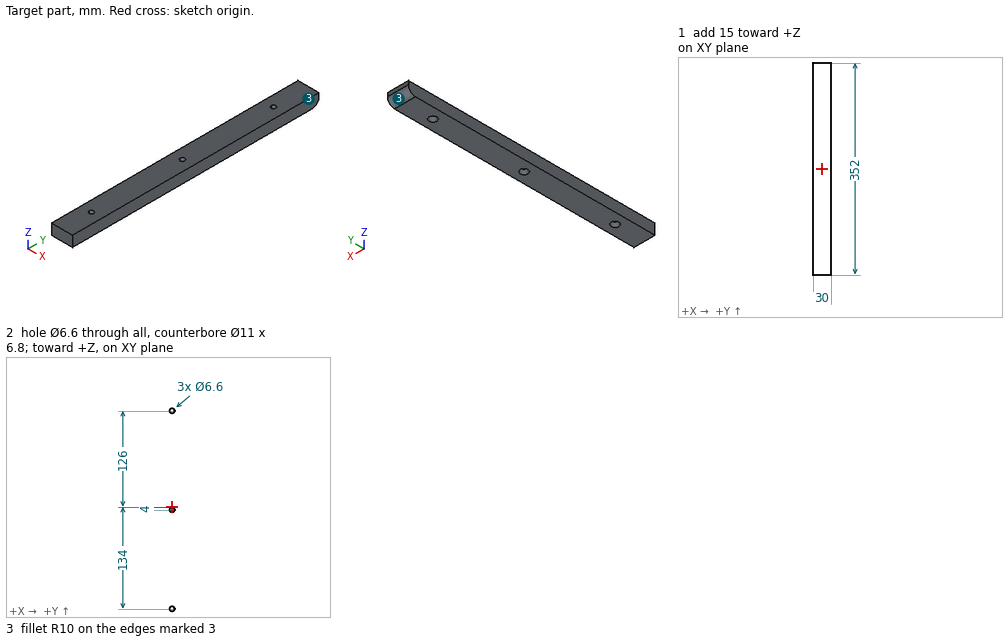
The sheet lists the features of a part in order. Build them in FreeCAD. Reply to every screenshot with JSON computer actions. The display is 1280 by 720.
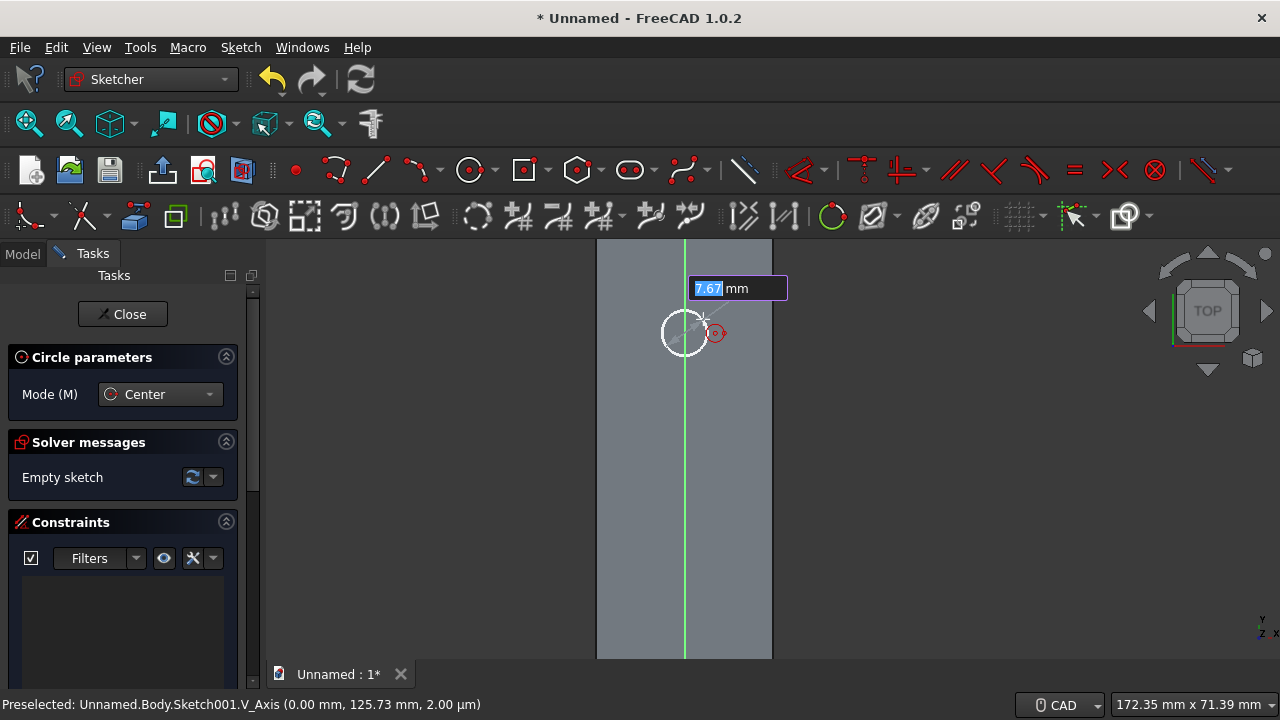
{"action": "type", "text": "6.6"}
{"action": "key", "text": "Return"}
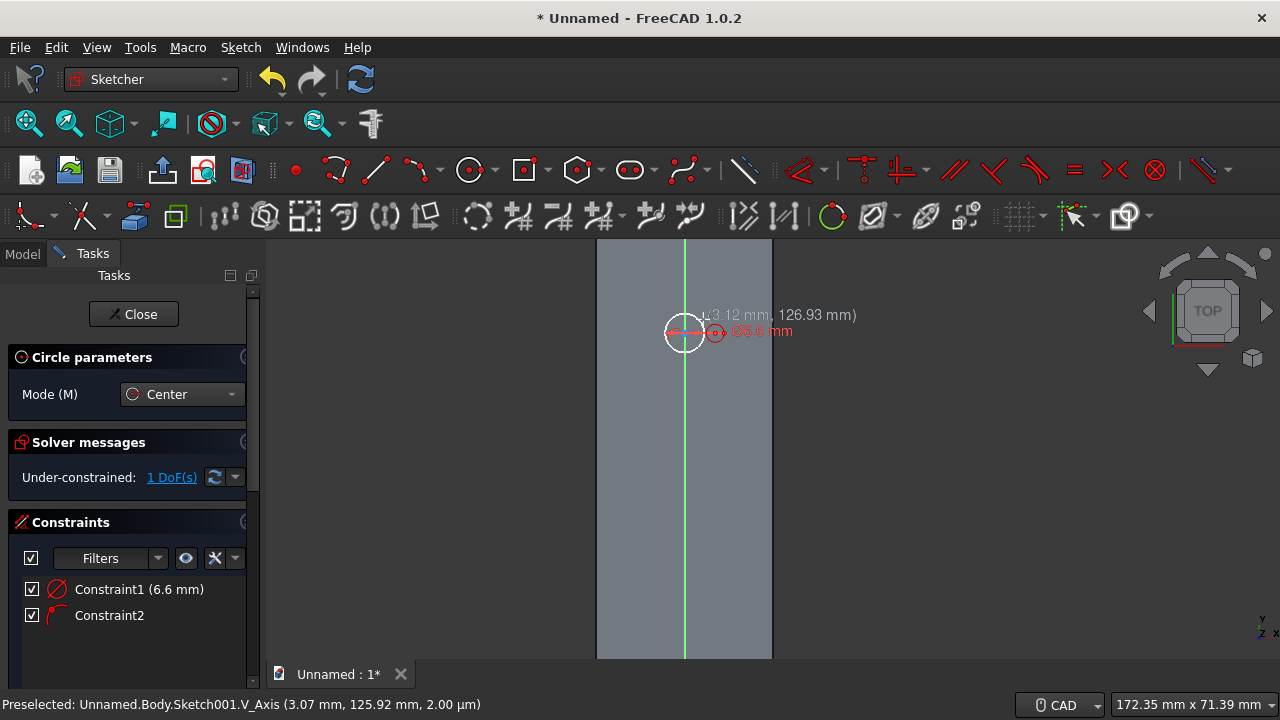
{"action": "scroll", "coordinate": [708, 322], "scroll_direction": "down", "scroll_amount": 9}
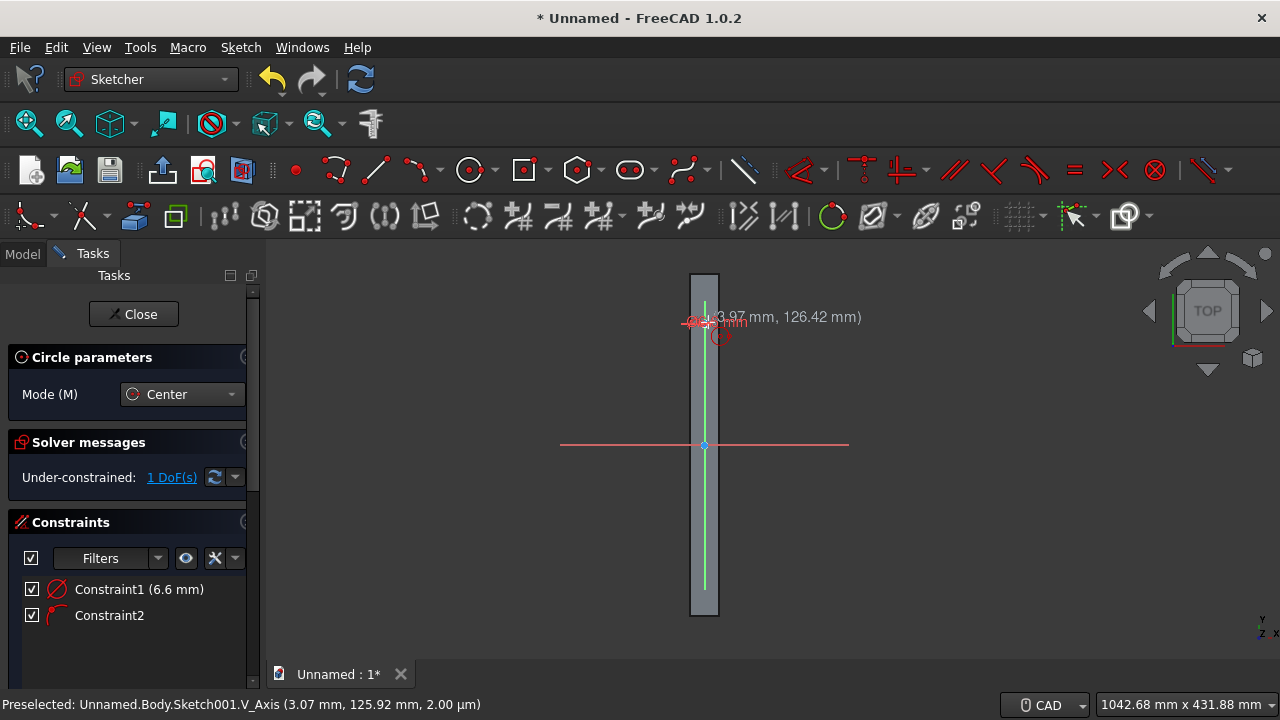
{"action": "scroll", "coordinate": [705, 449], "scroll_direction": "up", "scroll_amount": 10}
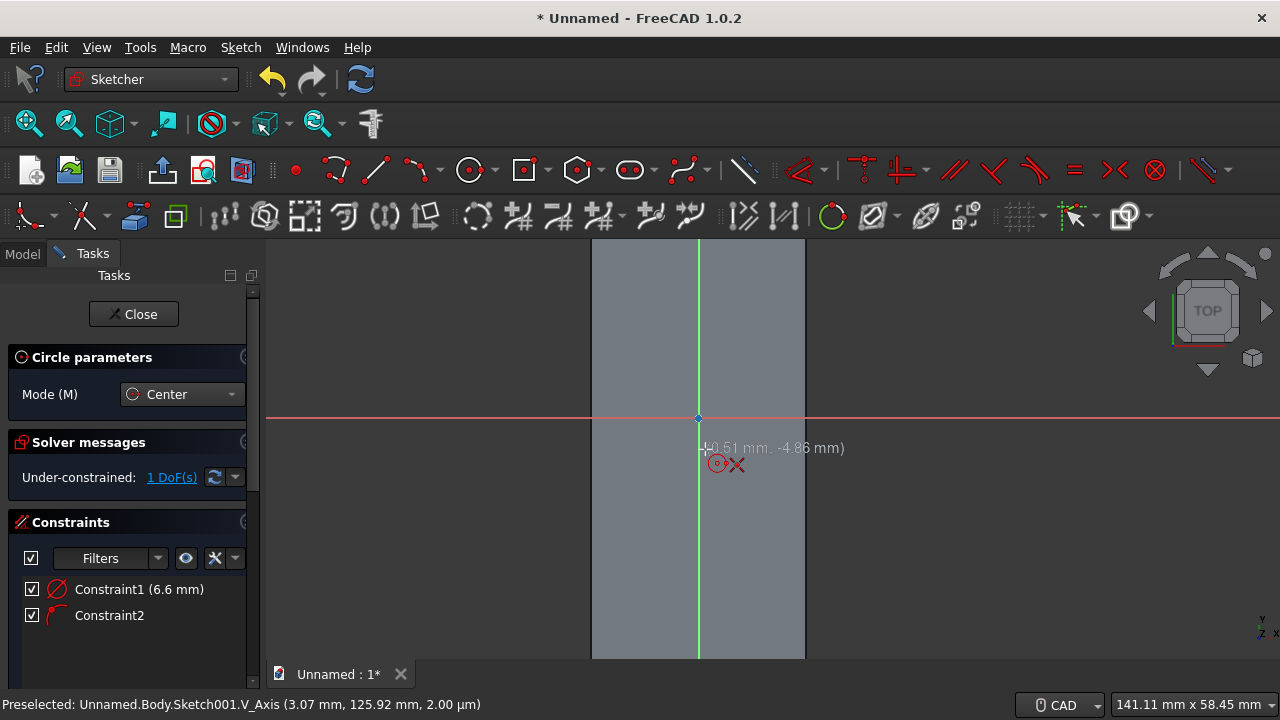
{"action": "left_click", "coordinate": [699, 447]}
{"action": "mouse_move", "coordinate": [715, 464]}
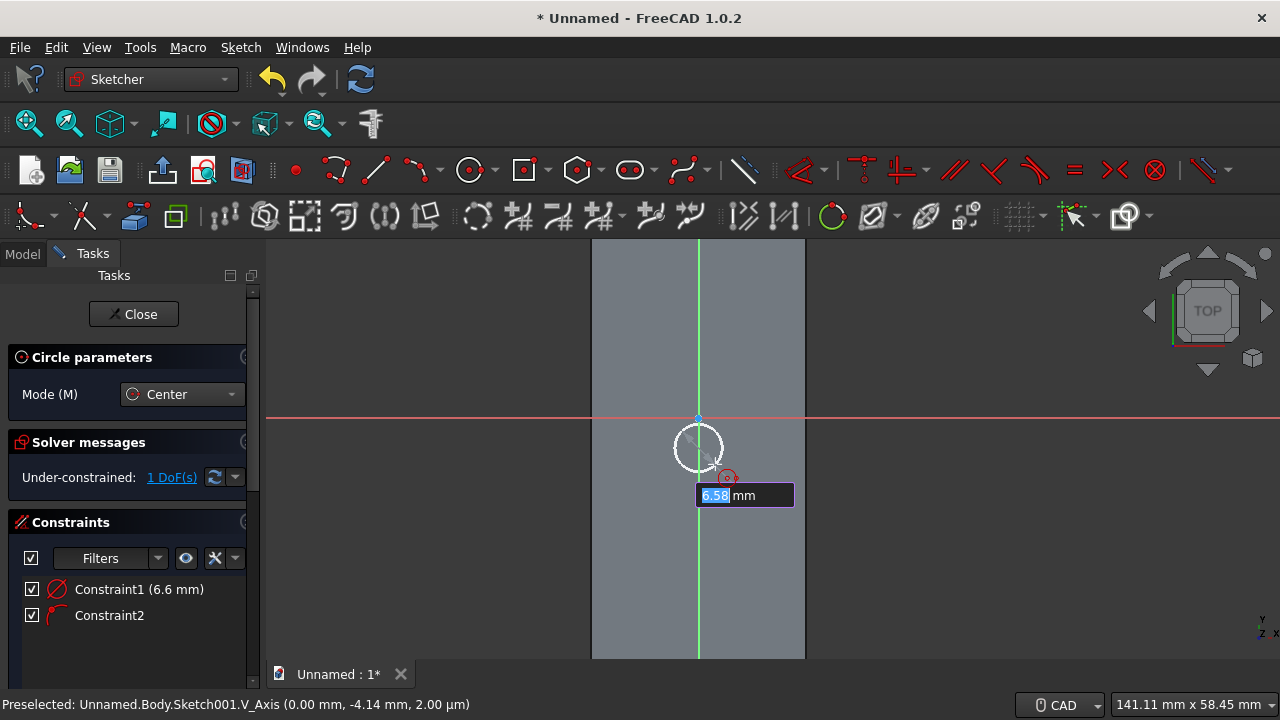
{"action": "type", "text": "6.6"}
{"action": "key", "text": "Return"}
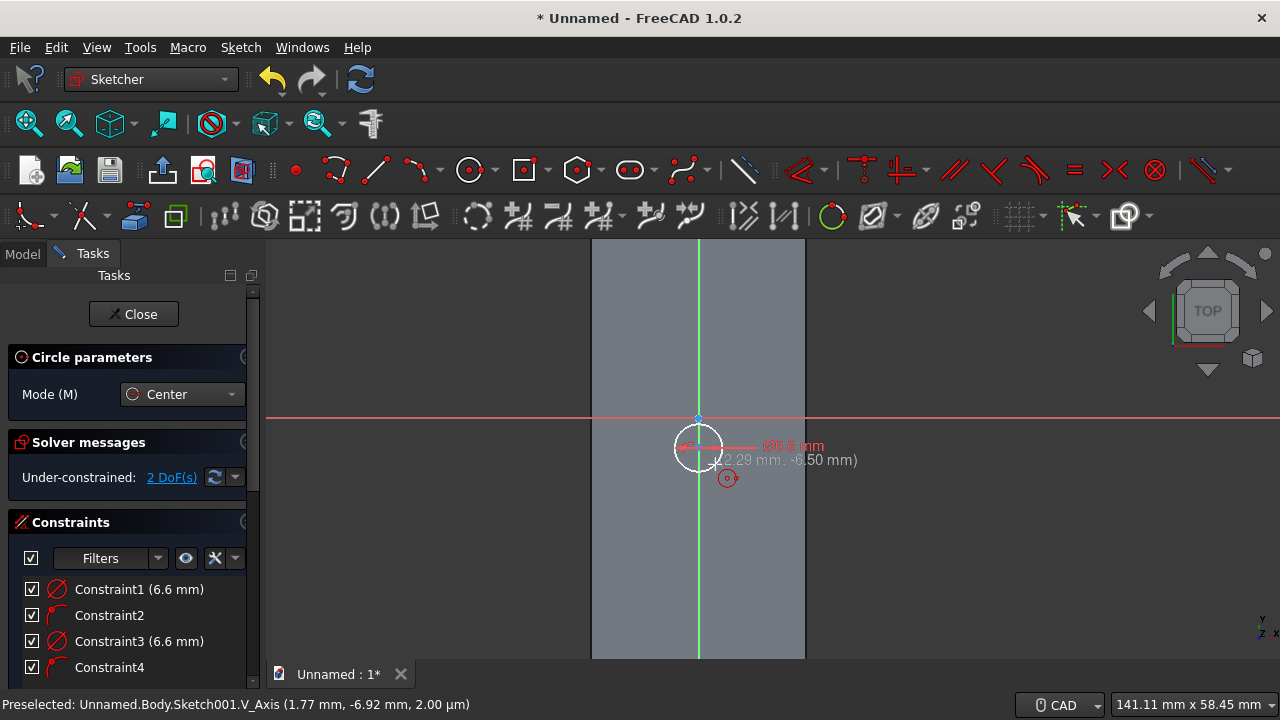
{"action": "scroll", "coordinate": [705, 449], "scroll_direction": "down", "scroll_amount": 10}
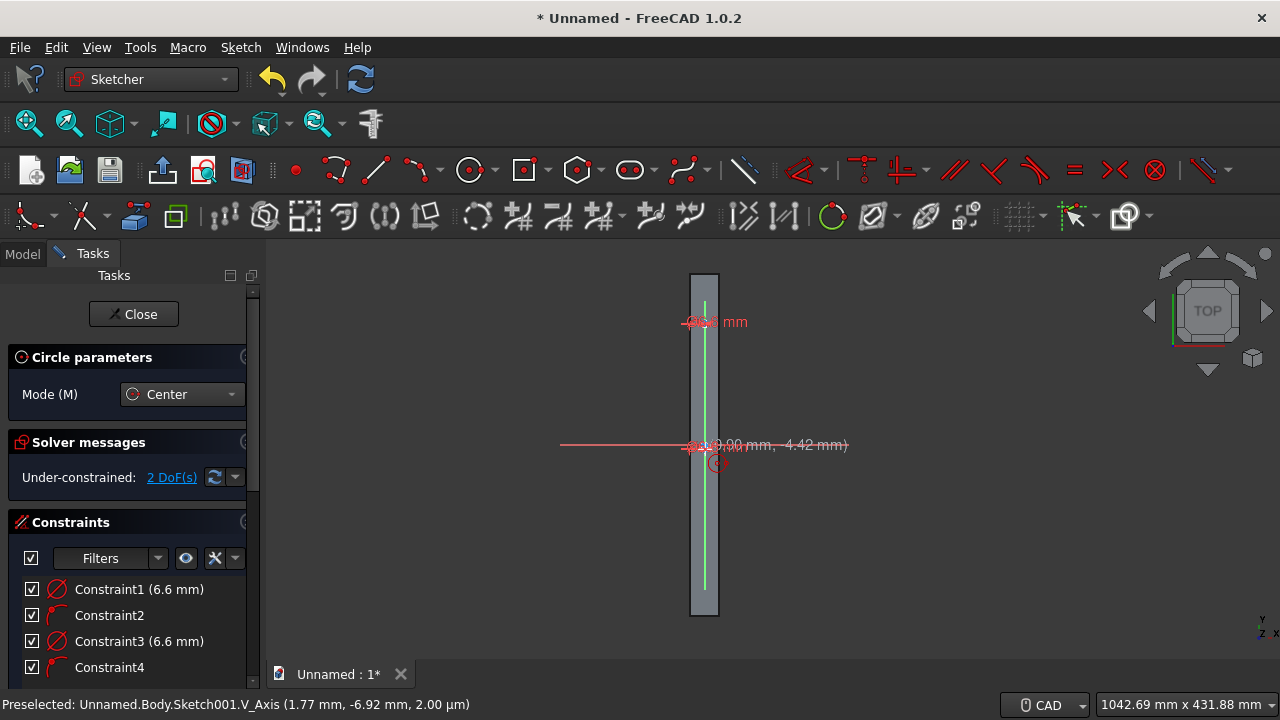
{"action": "scroll", "coordinate": [705, 576], "scroll_direction": "up", "scroll_amount": 10}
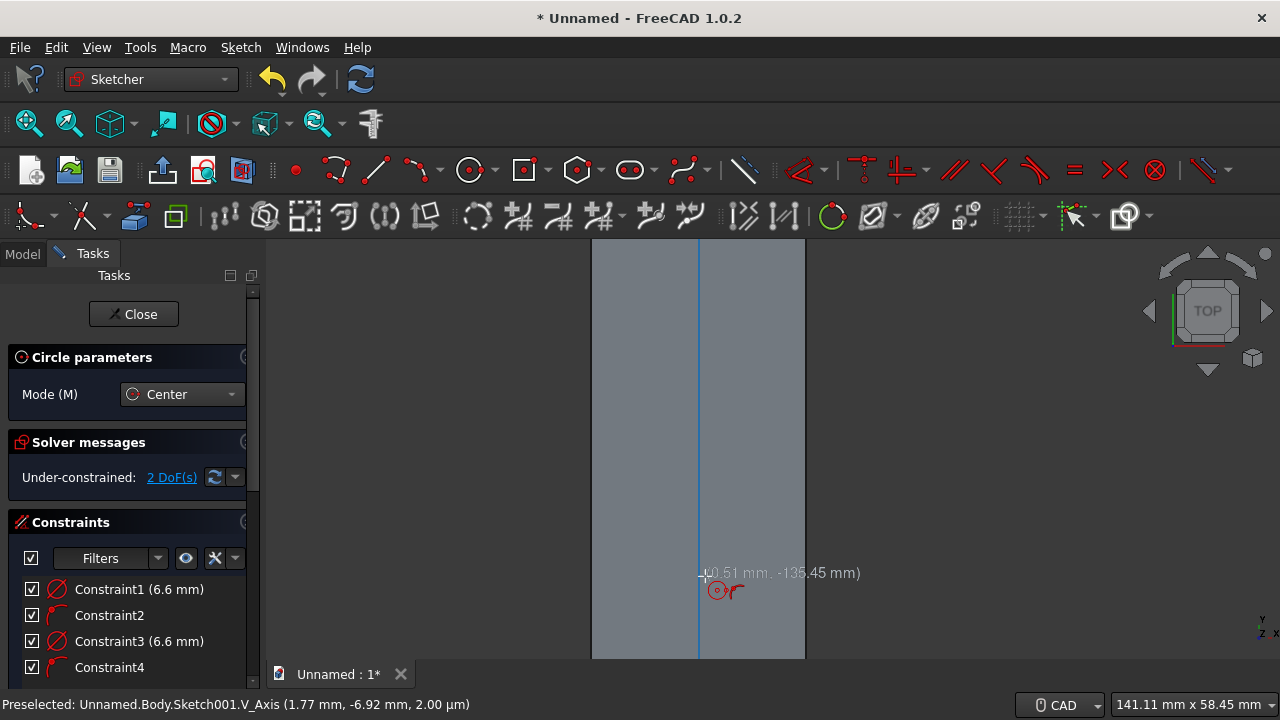
{"action": "scroll", "coordinate": [705, 577], "scroll_direction": "down", "scroll_amount": 10}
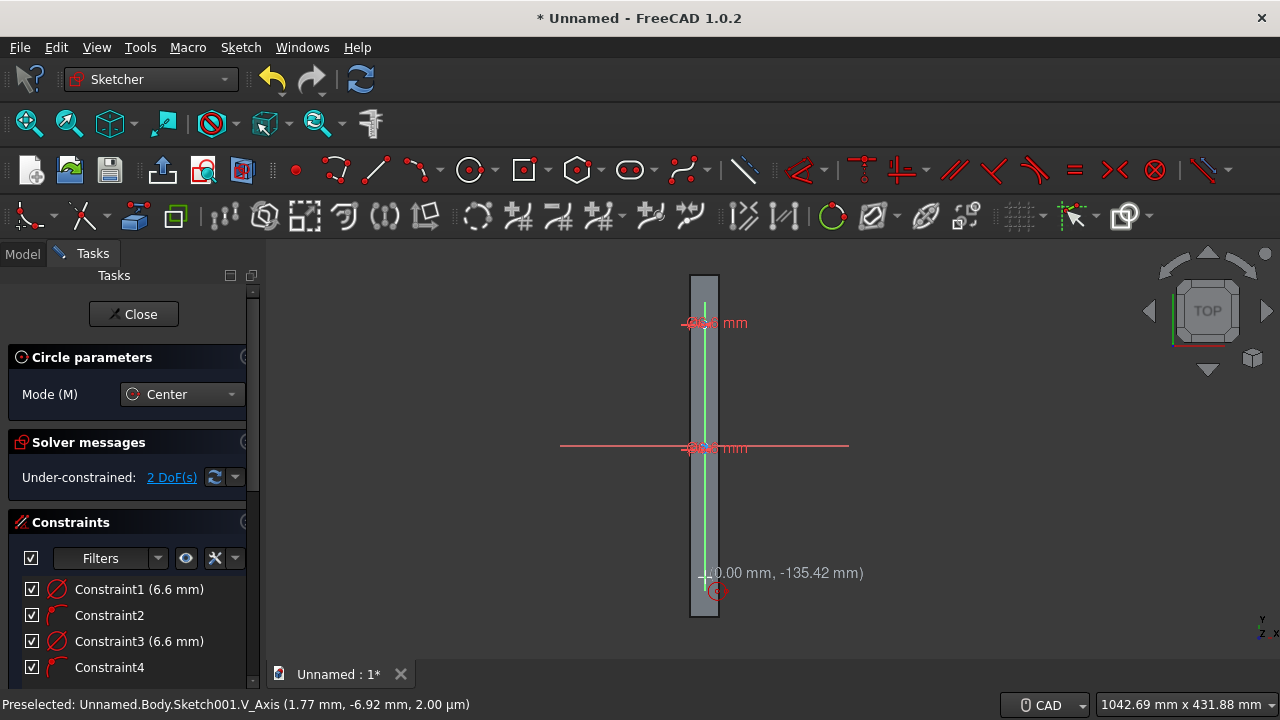
{"action": "left_click", "coordinate": [705, 576]}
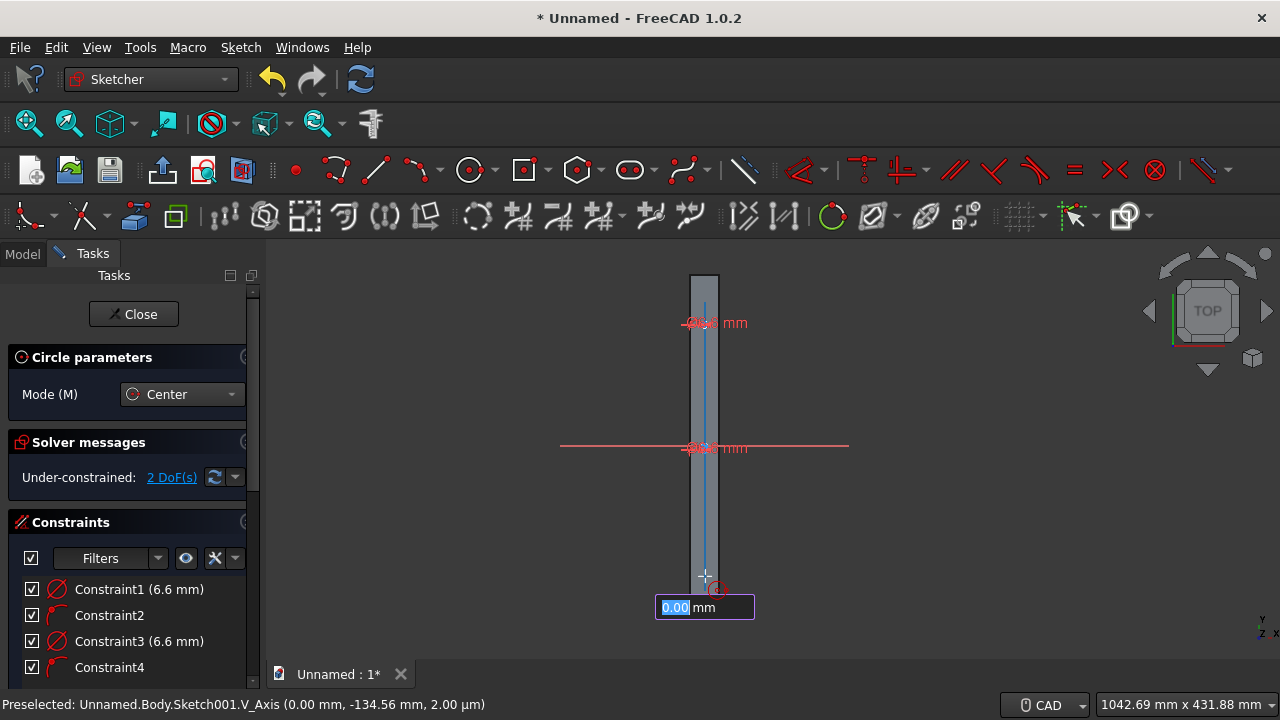
{"action": "scroll", "coordinate": [708, 575], "scroll_direction": "up", "scroll_amount": 9}
{"action": "mouse_move", "coordinate": [703, 573]}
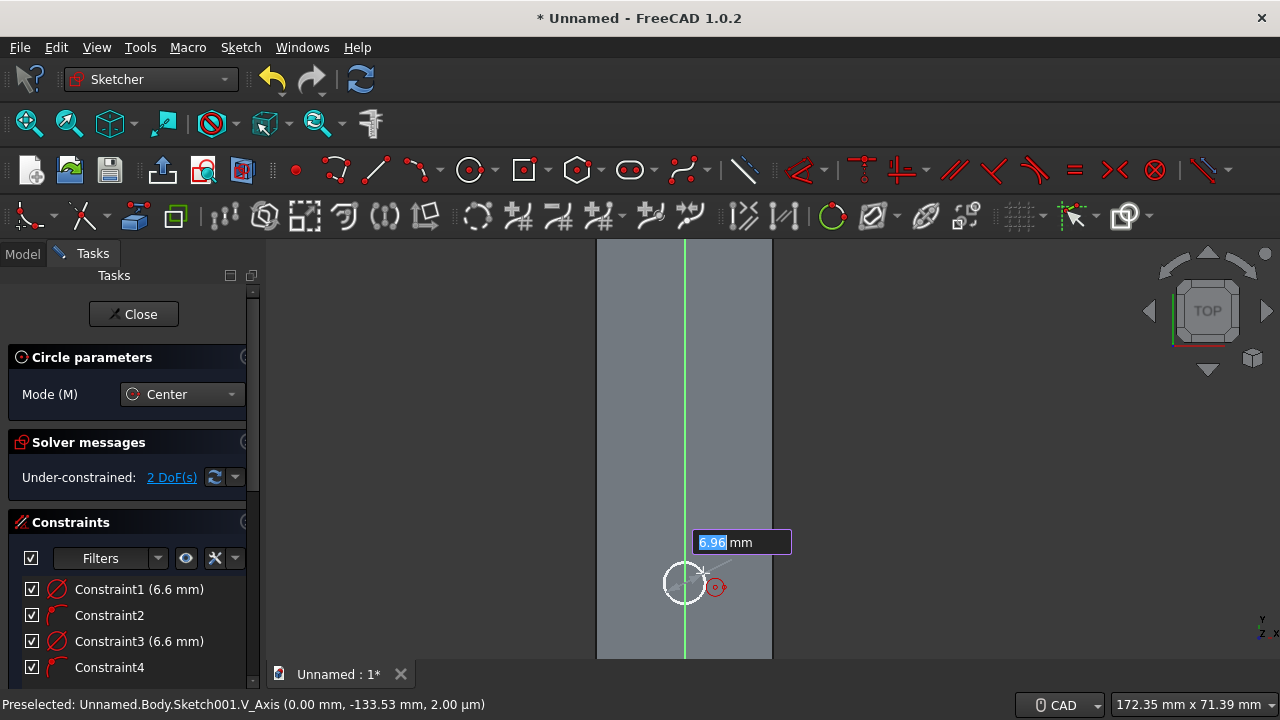
{"action": "type", "text": "6.6"}
{"action": "key", "text": "Return"}
{"action": "key", "text": "Escape"}